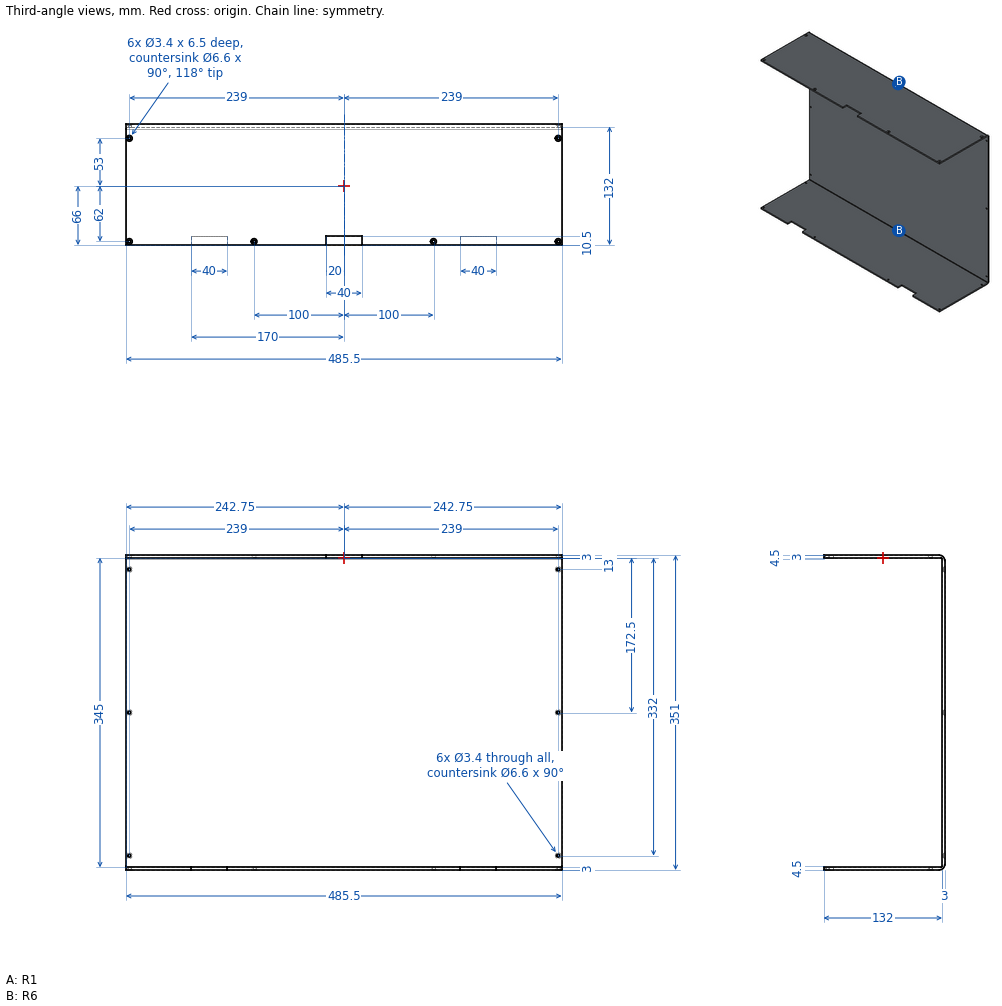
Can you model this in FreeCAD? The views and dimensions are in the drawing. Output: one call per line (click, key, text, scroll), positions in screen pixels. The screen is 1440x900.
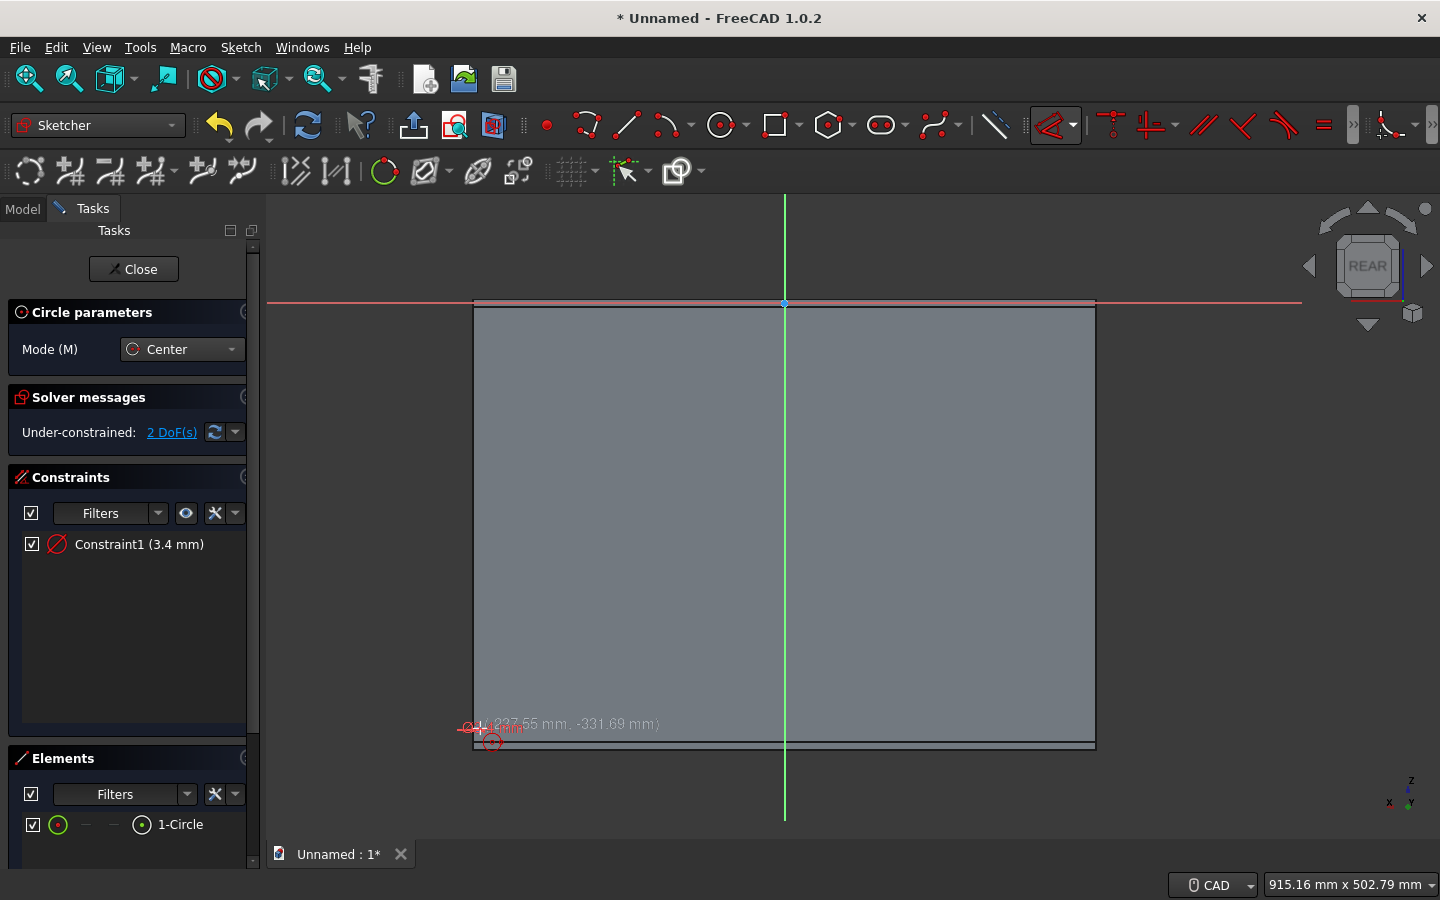
scroll(478, 525, up, 12)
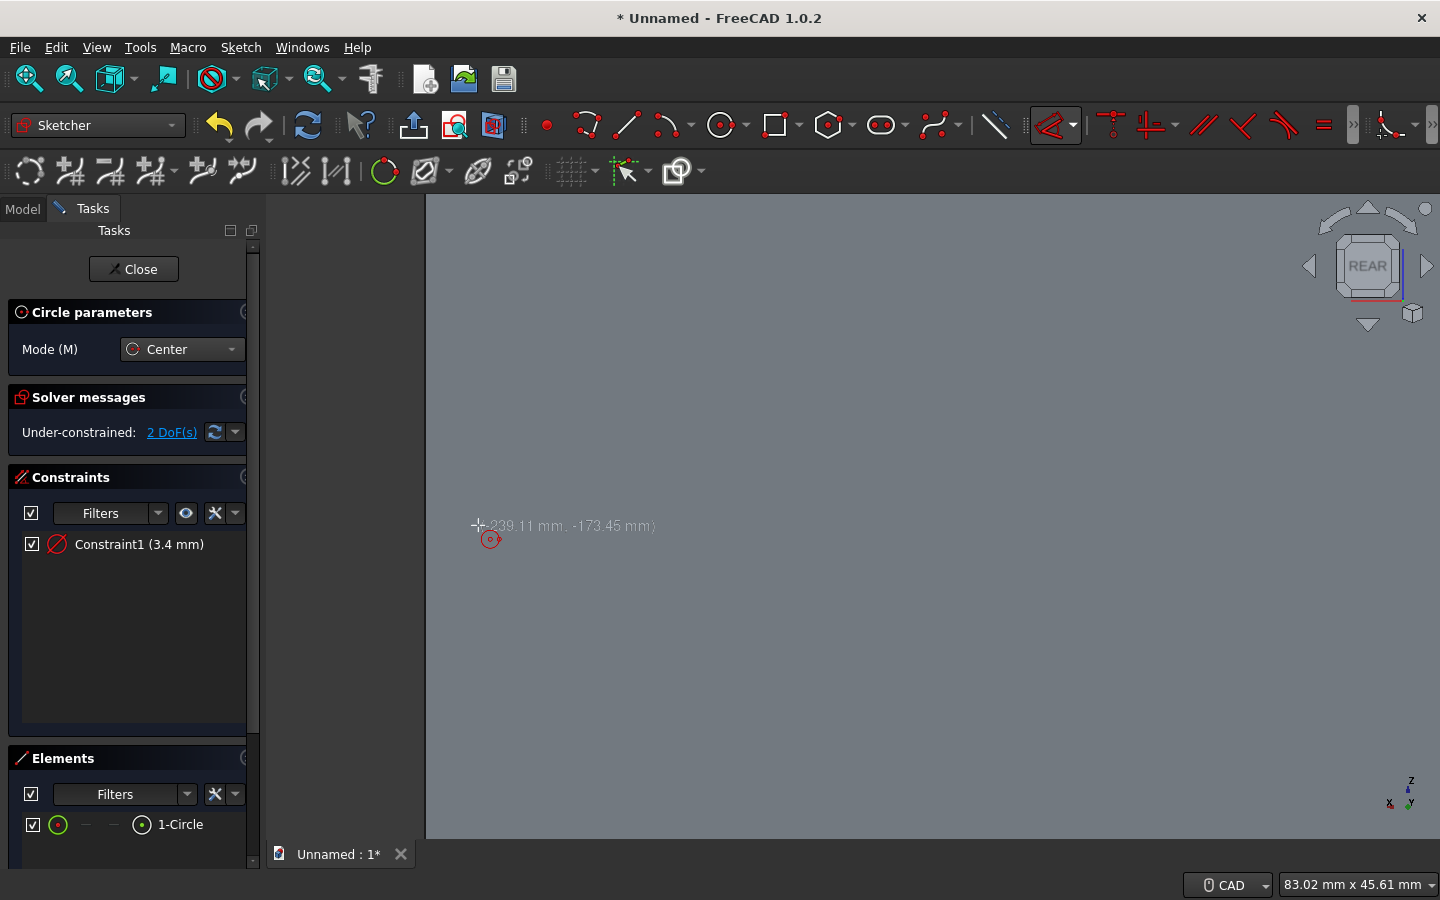
scroll(478, 524, down, 12)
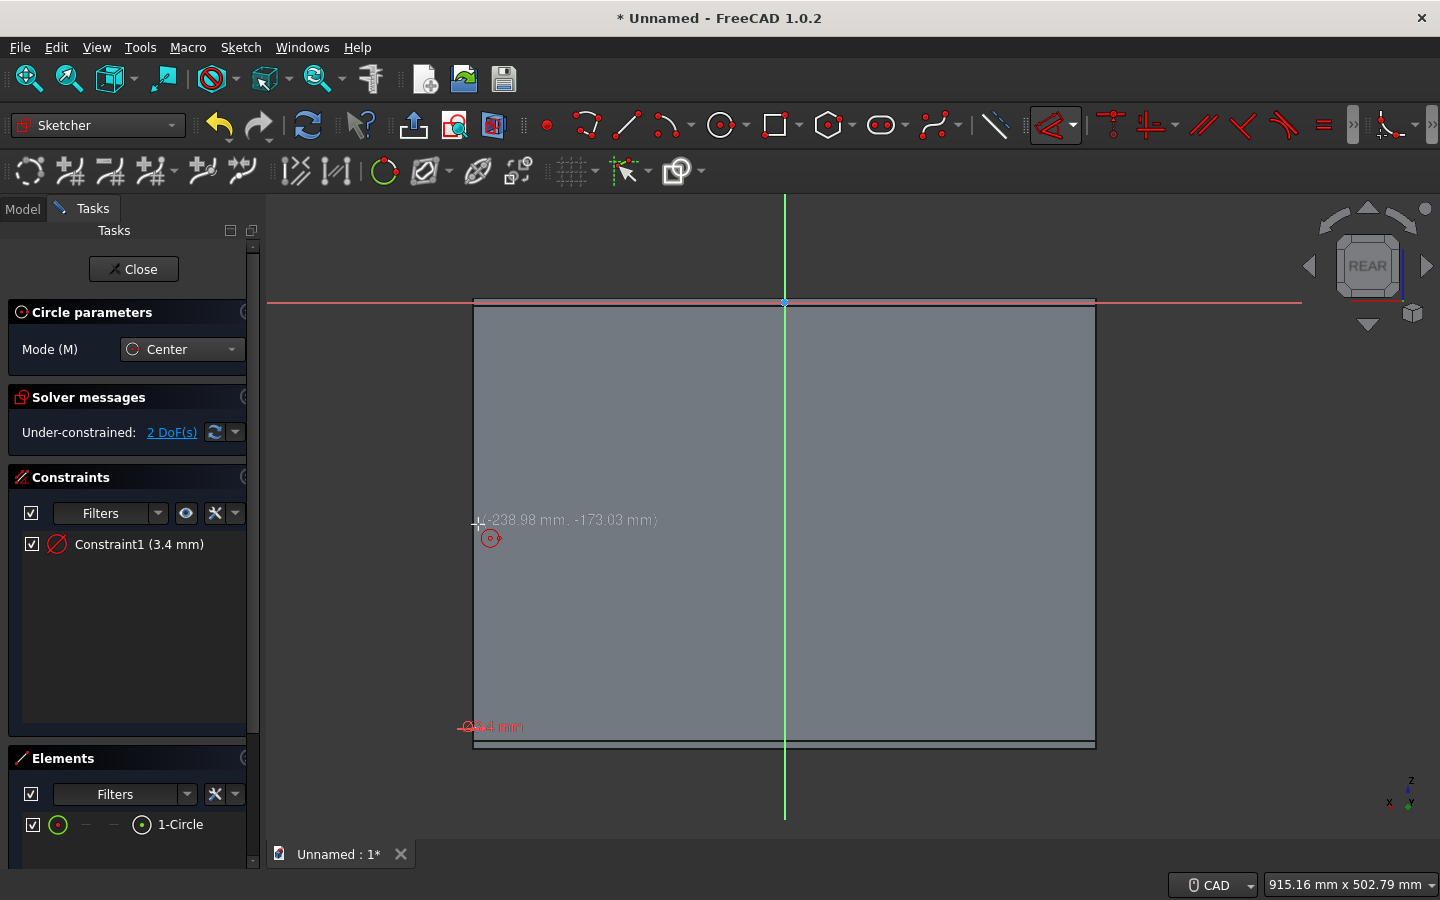
click(478, 524)
move(480, 522)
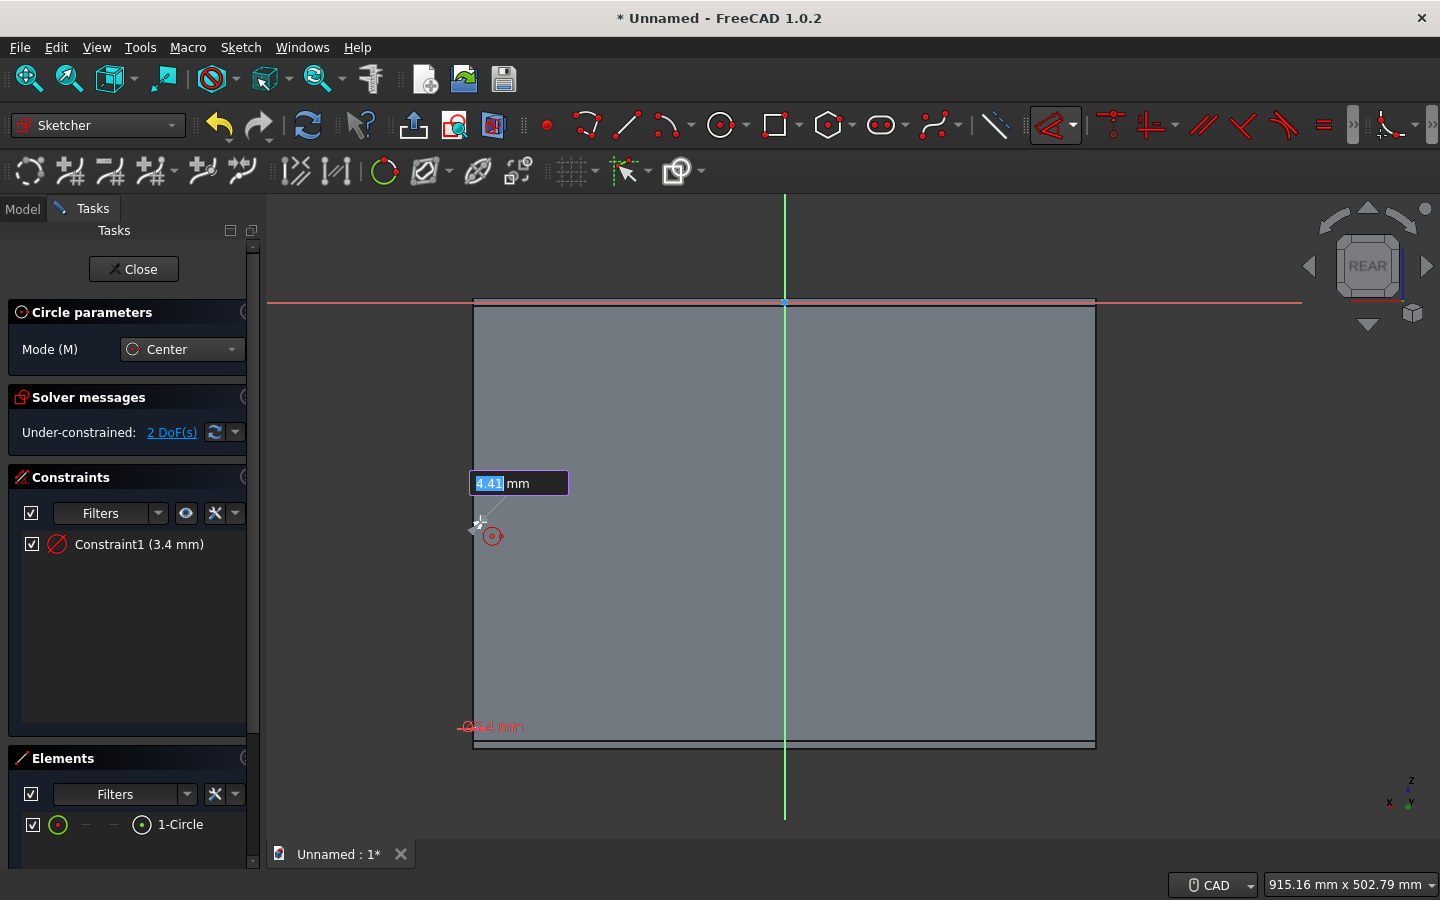
text(3.4)
key(Return)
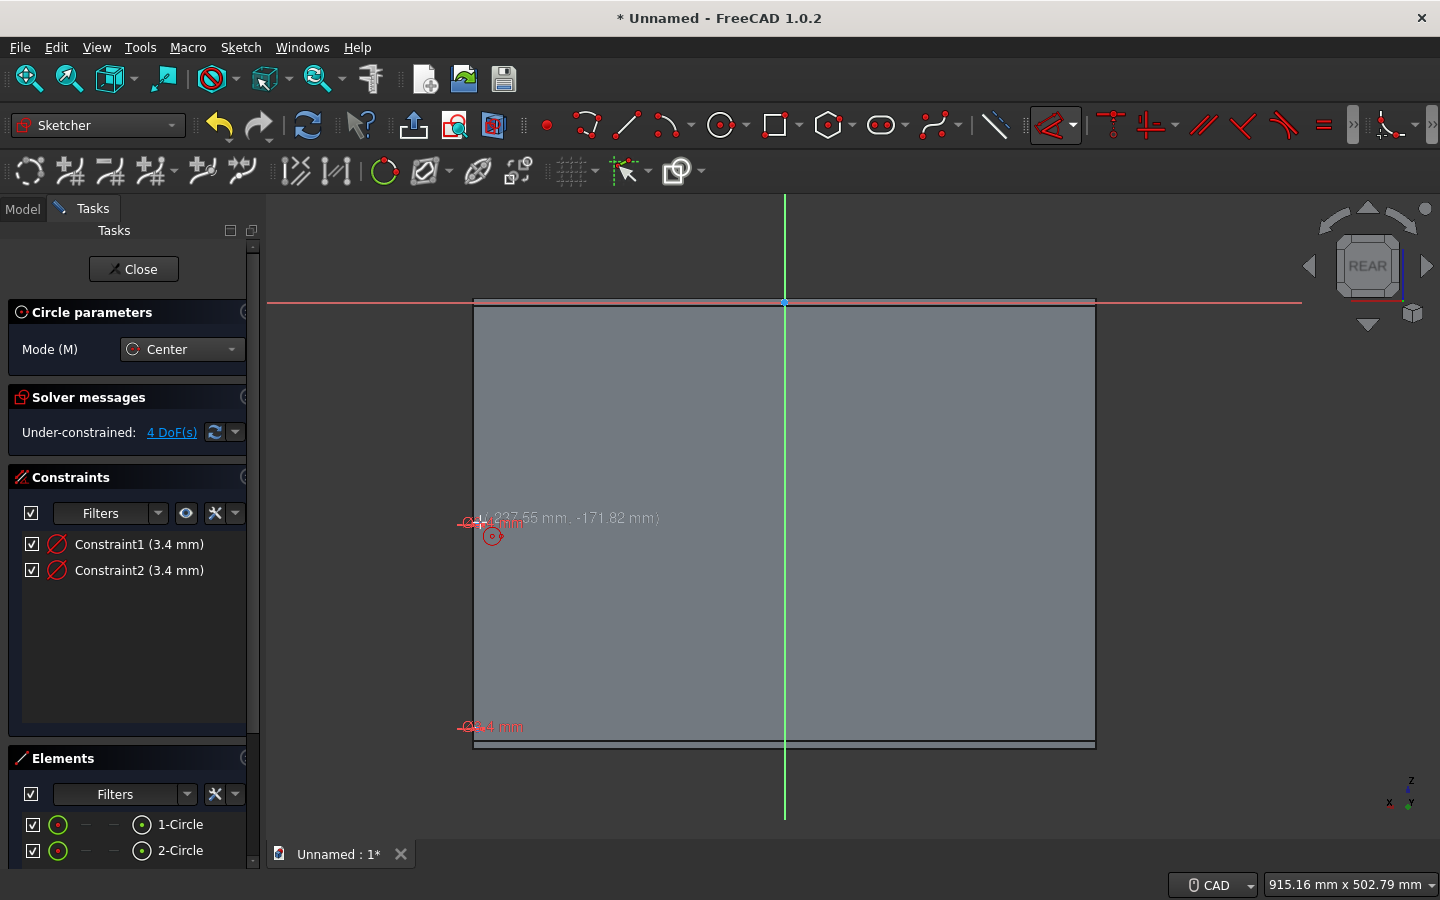
scroll(478, 319, up, 12)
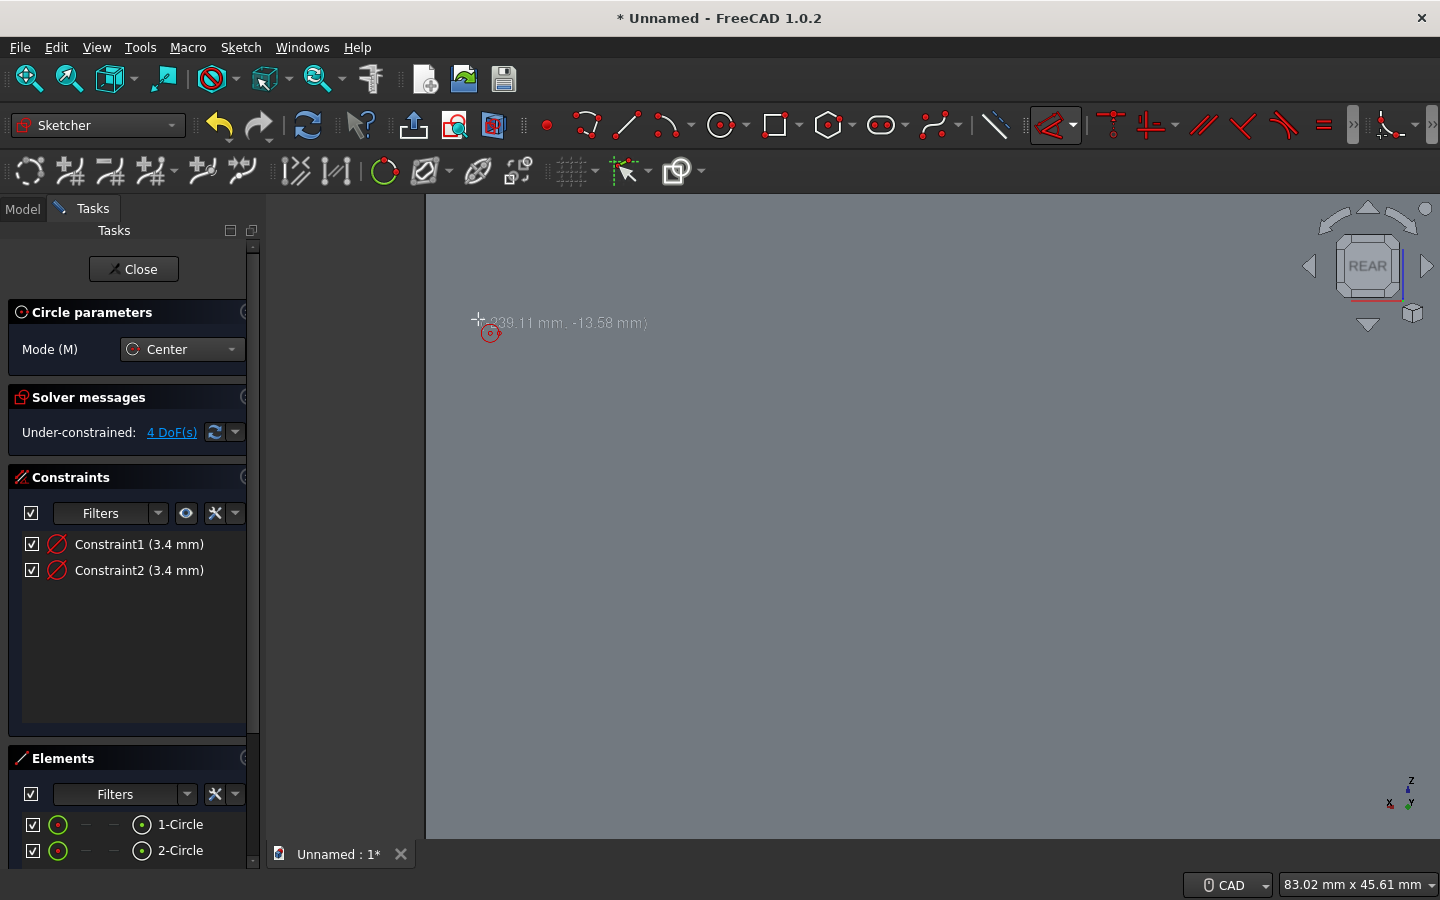
scroll(478, 319, down, 12)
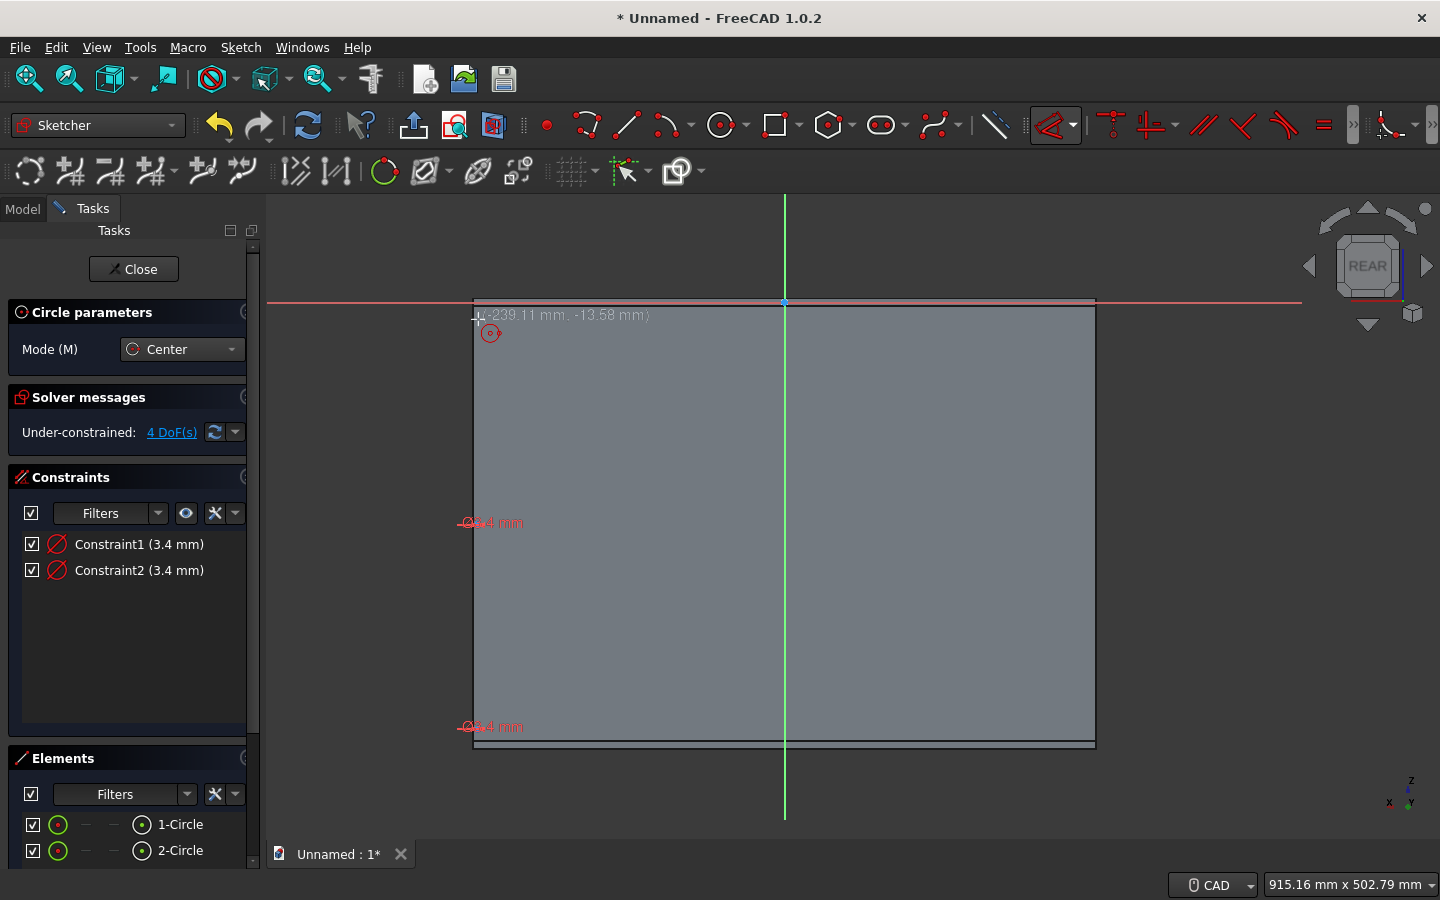
click(478, 319)
move(480, 318)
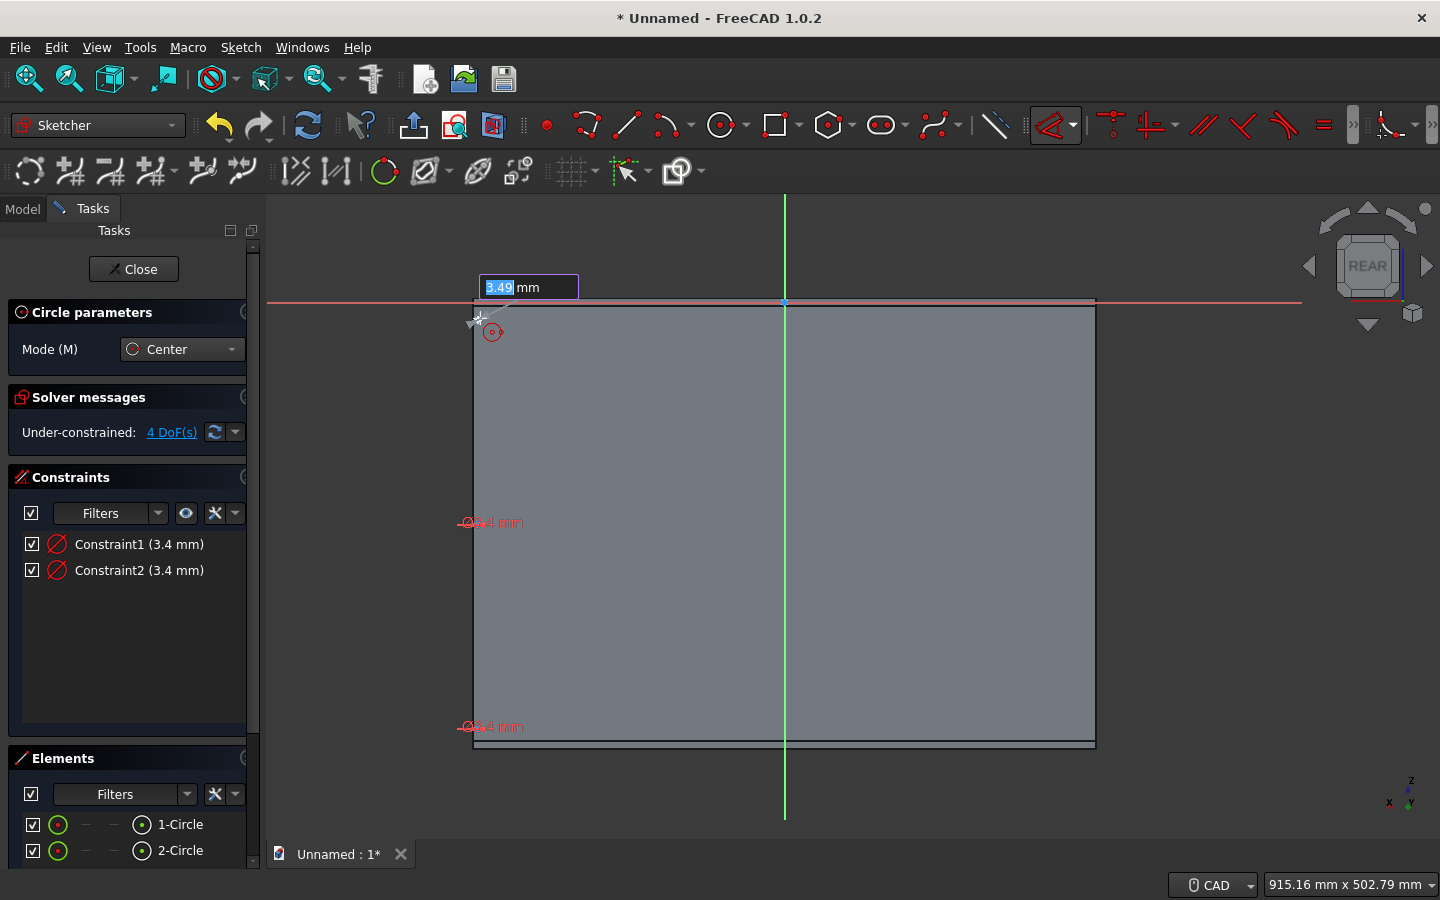
text(3.4)
key(Return)